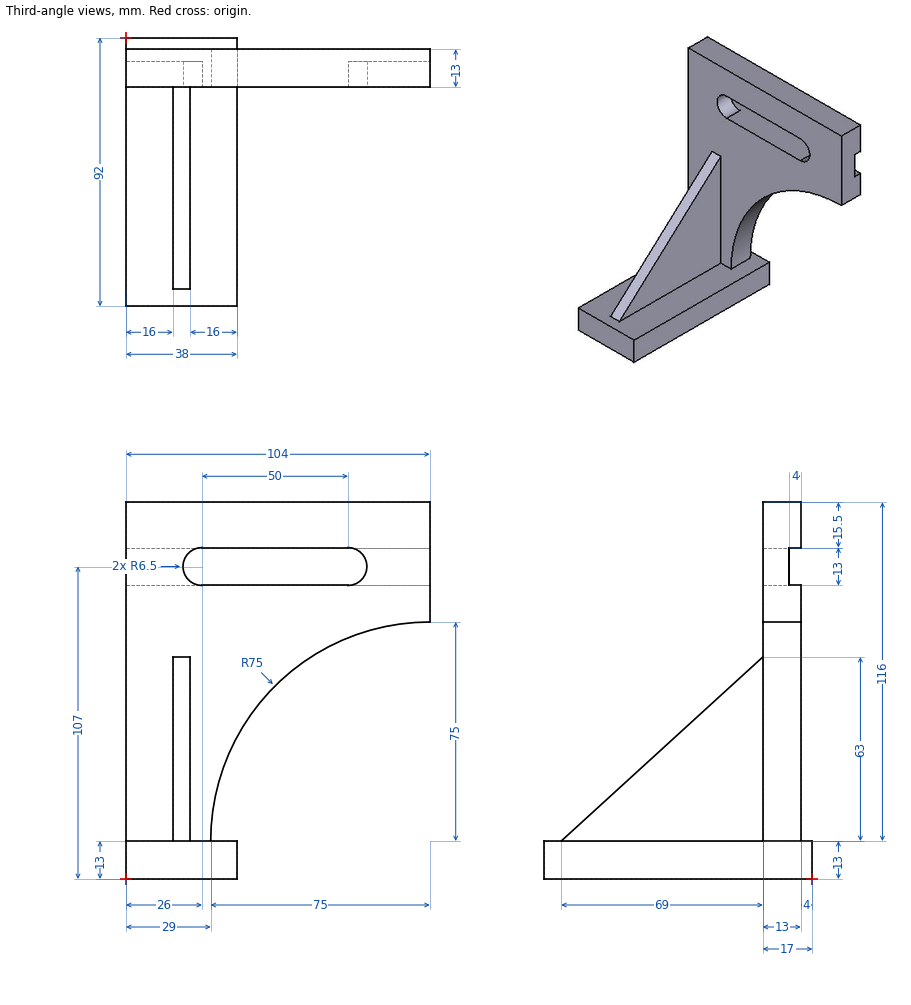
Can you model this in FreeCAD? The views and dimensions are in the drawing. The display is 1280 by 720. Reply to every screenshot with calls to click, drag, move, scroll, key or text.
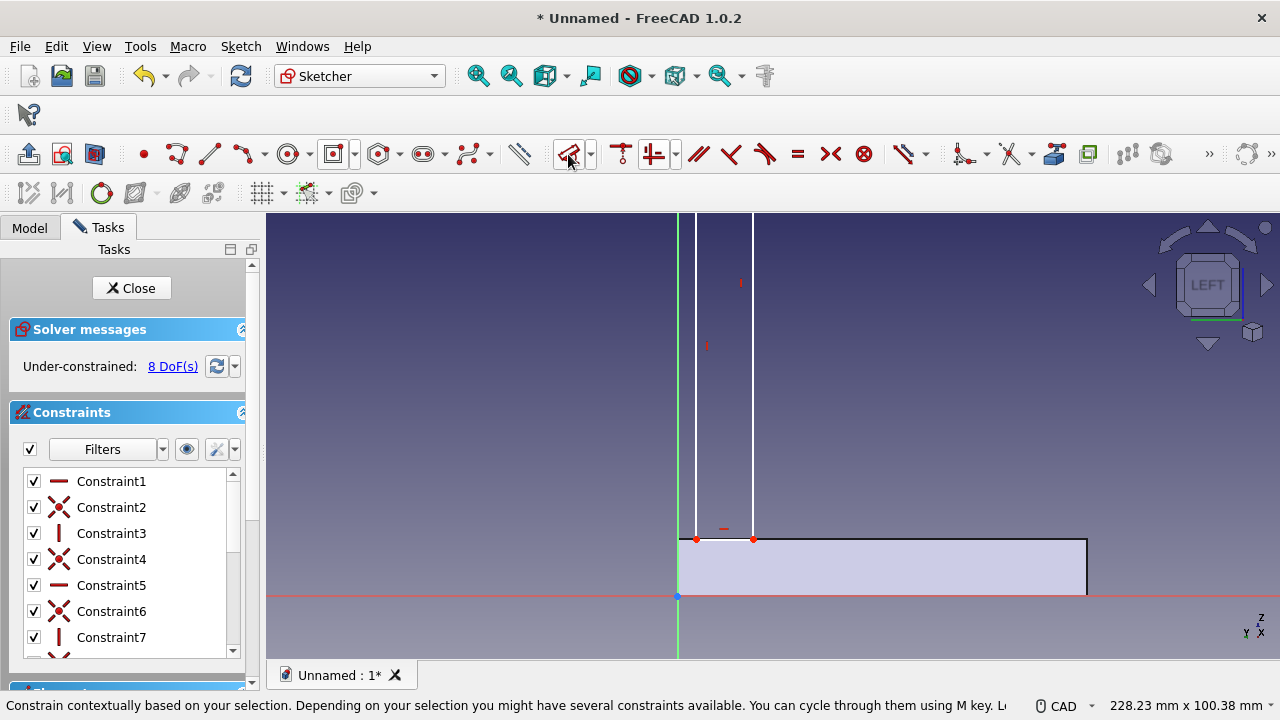
scroll(695, 539, down, 4)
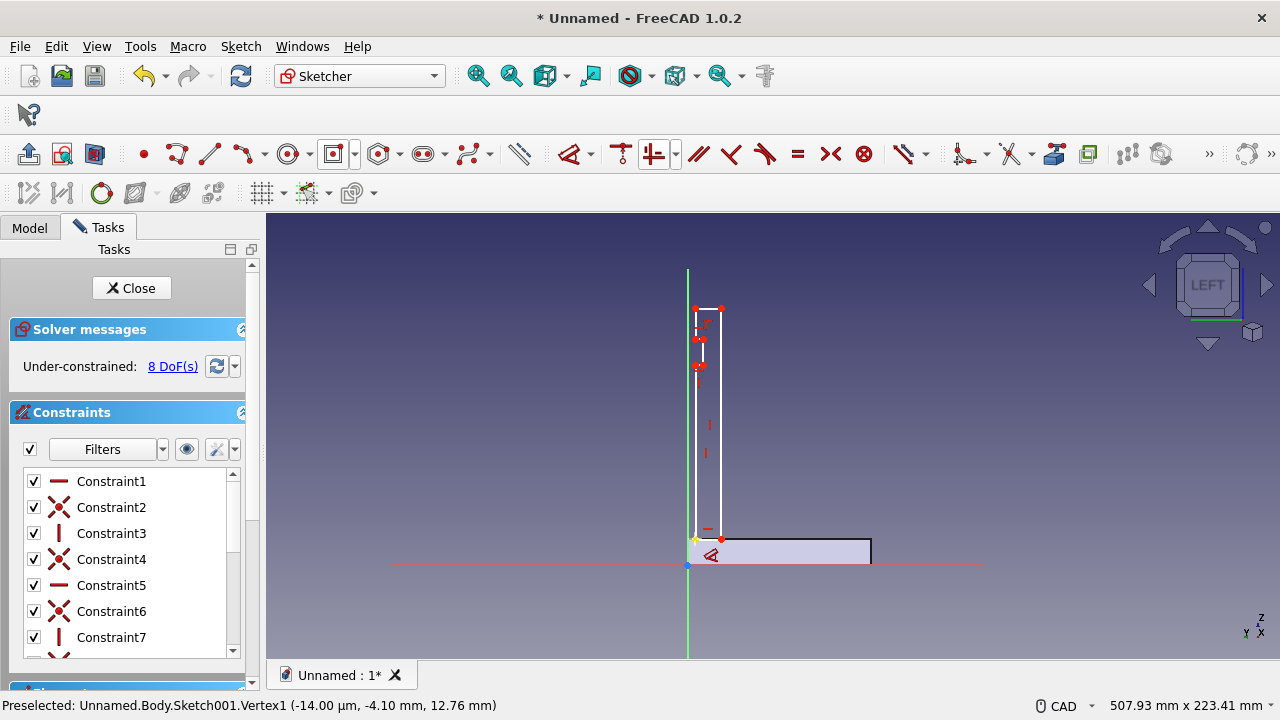
scroll(700, 339, up, 9)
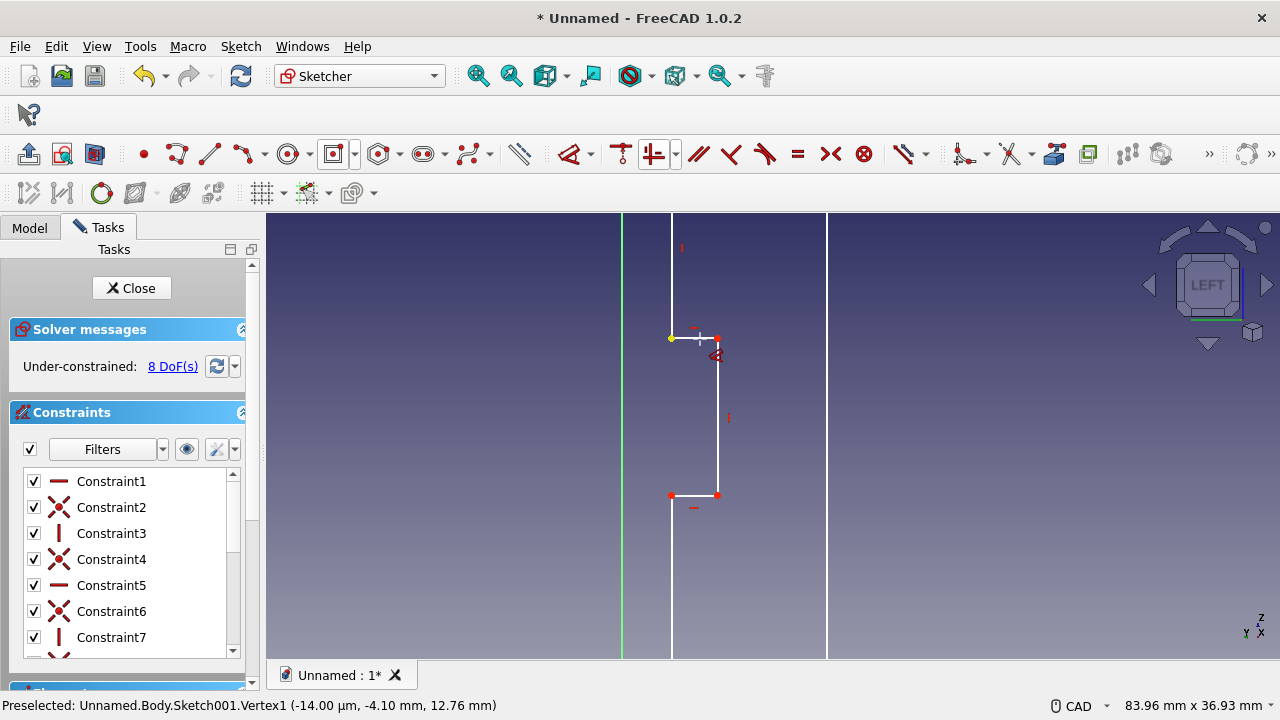
click(695, 338)
click(695, 304)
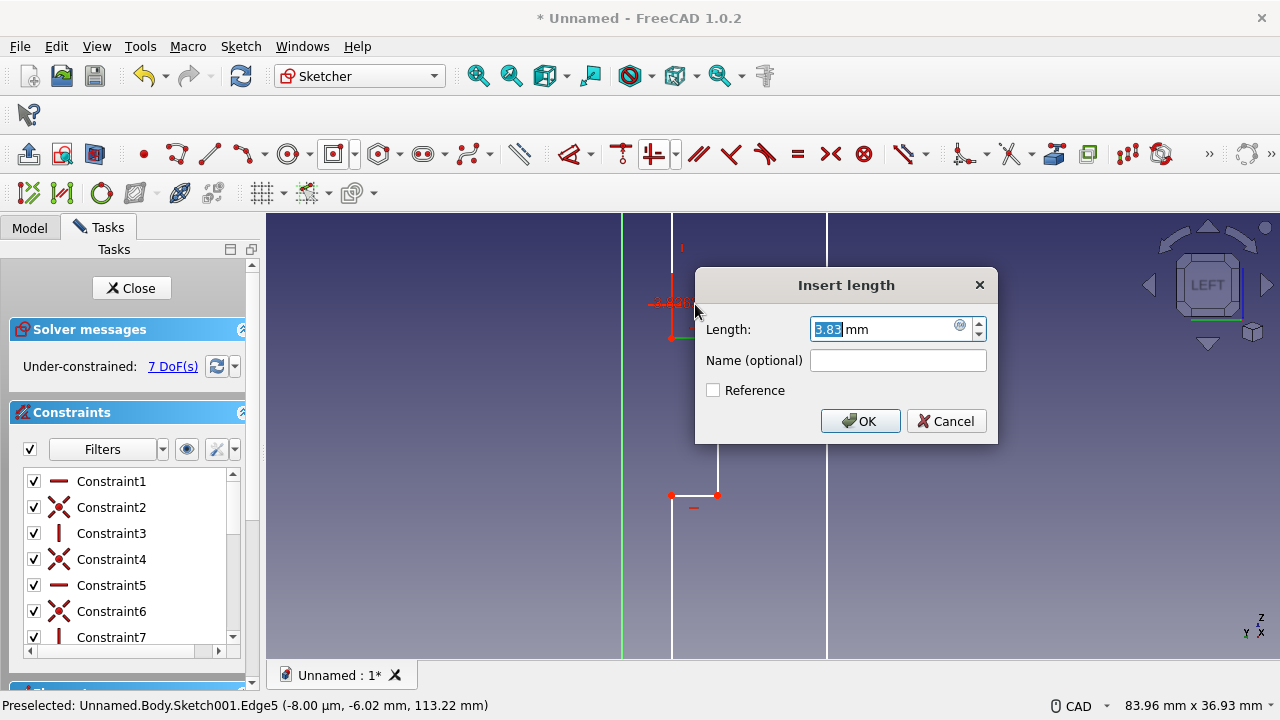
text(4)
key(Return)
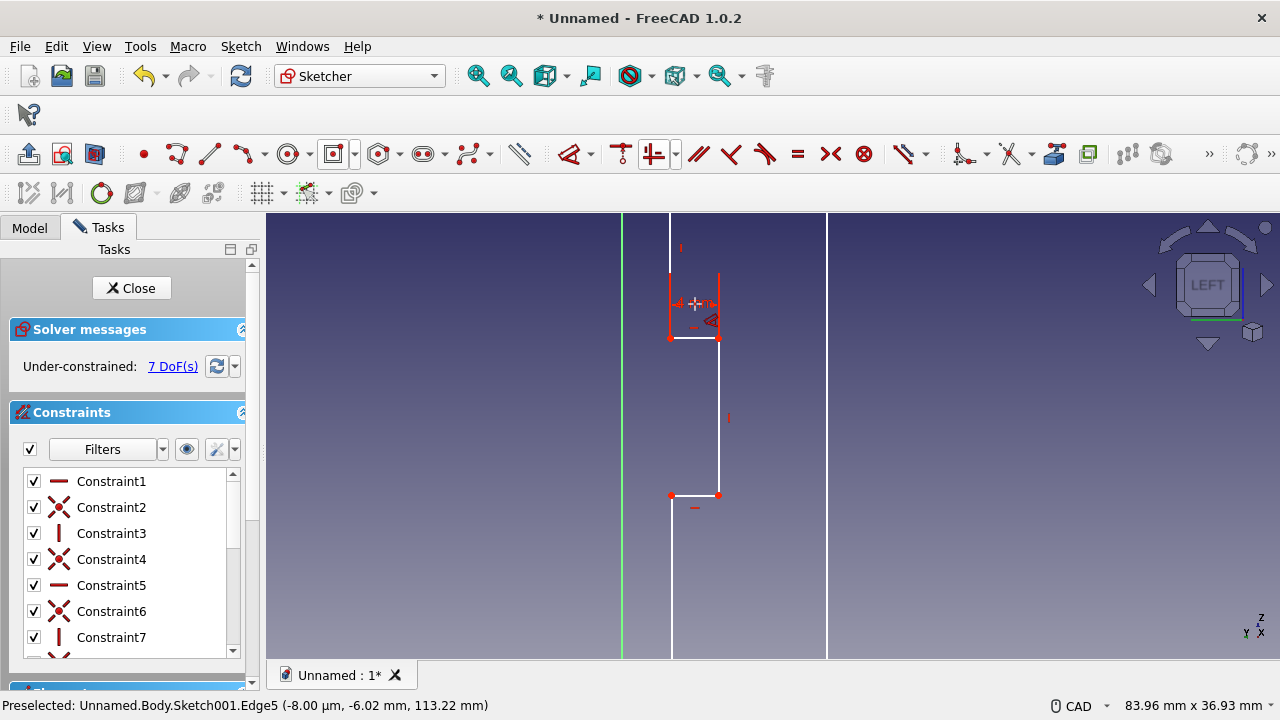
click(705, 496)
click(695, 462)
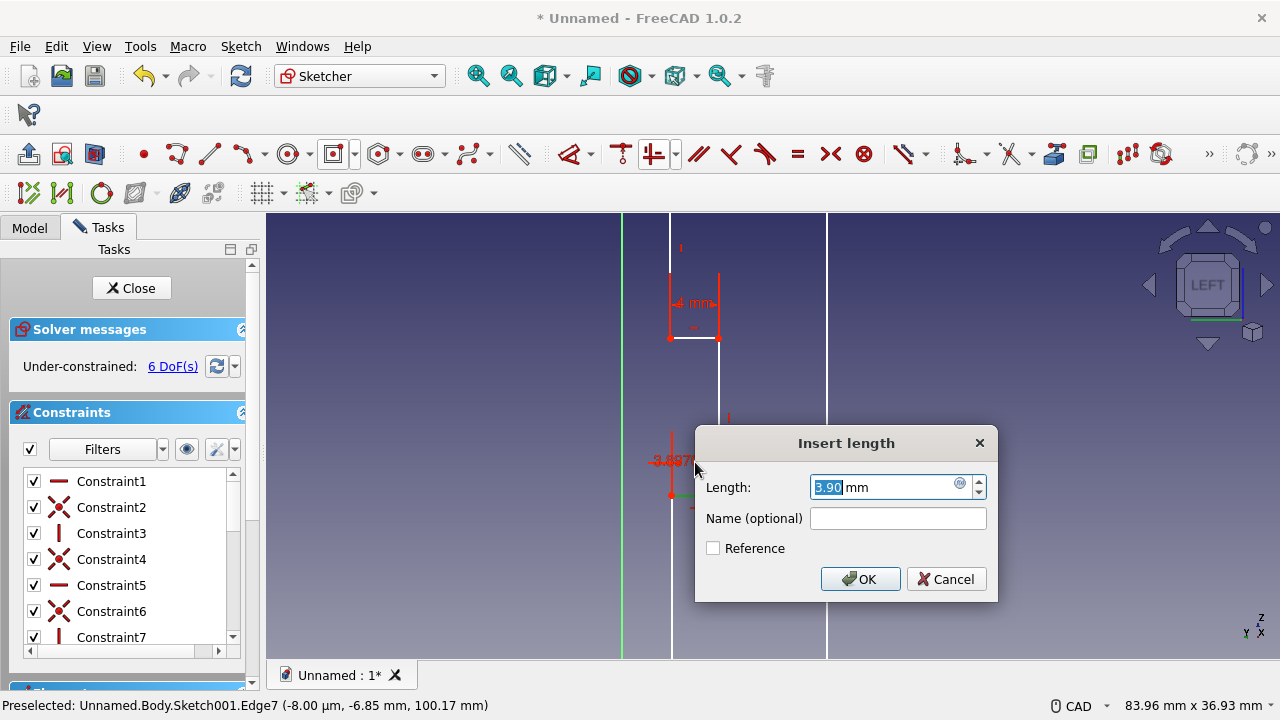
text(4)
key(Return)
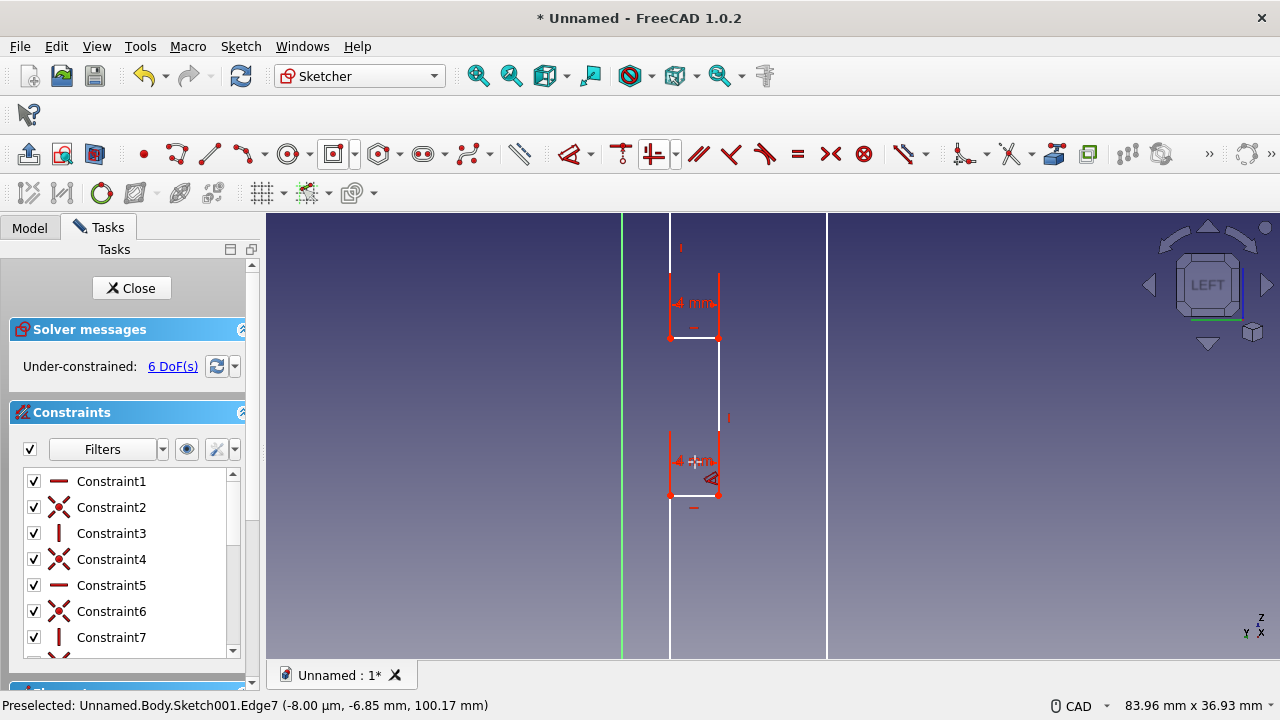
scroll(700, 339, down, 9)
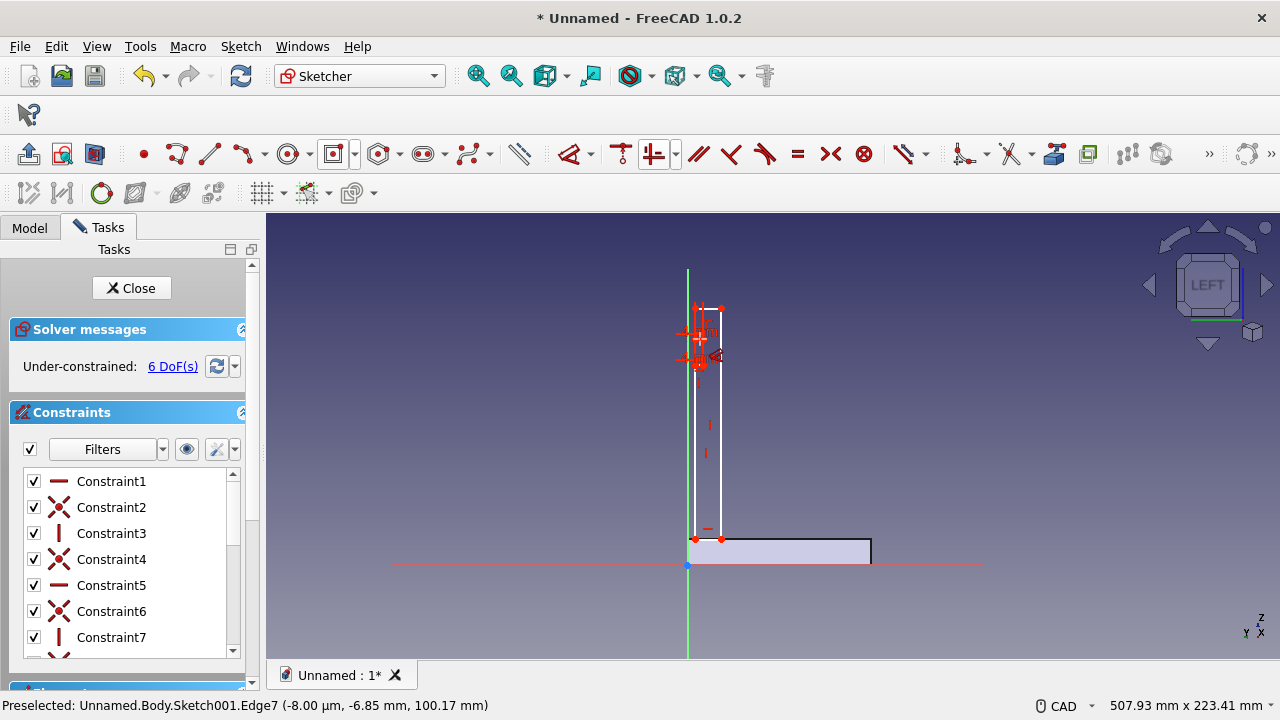
scroll(703, 540, up, 3)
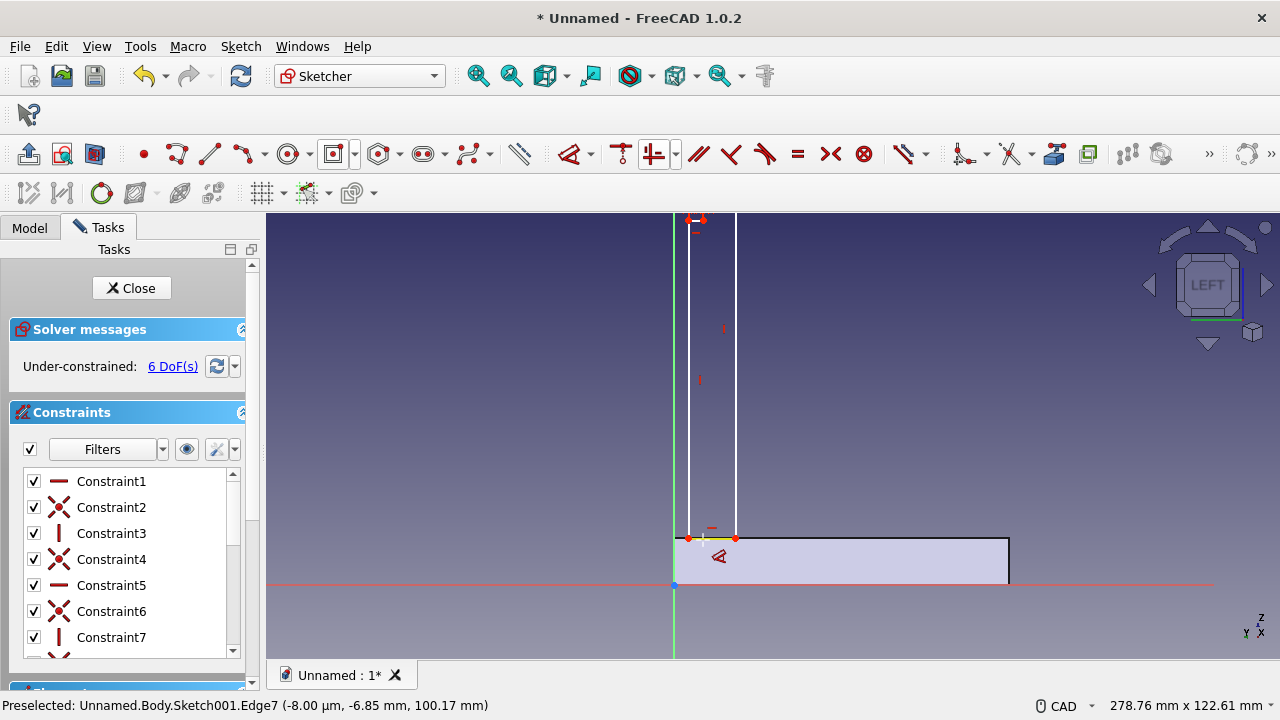
click(703, 539)
click(712, 505)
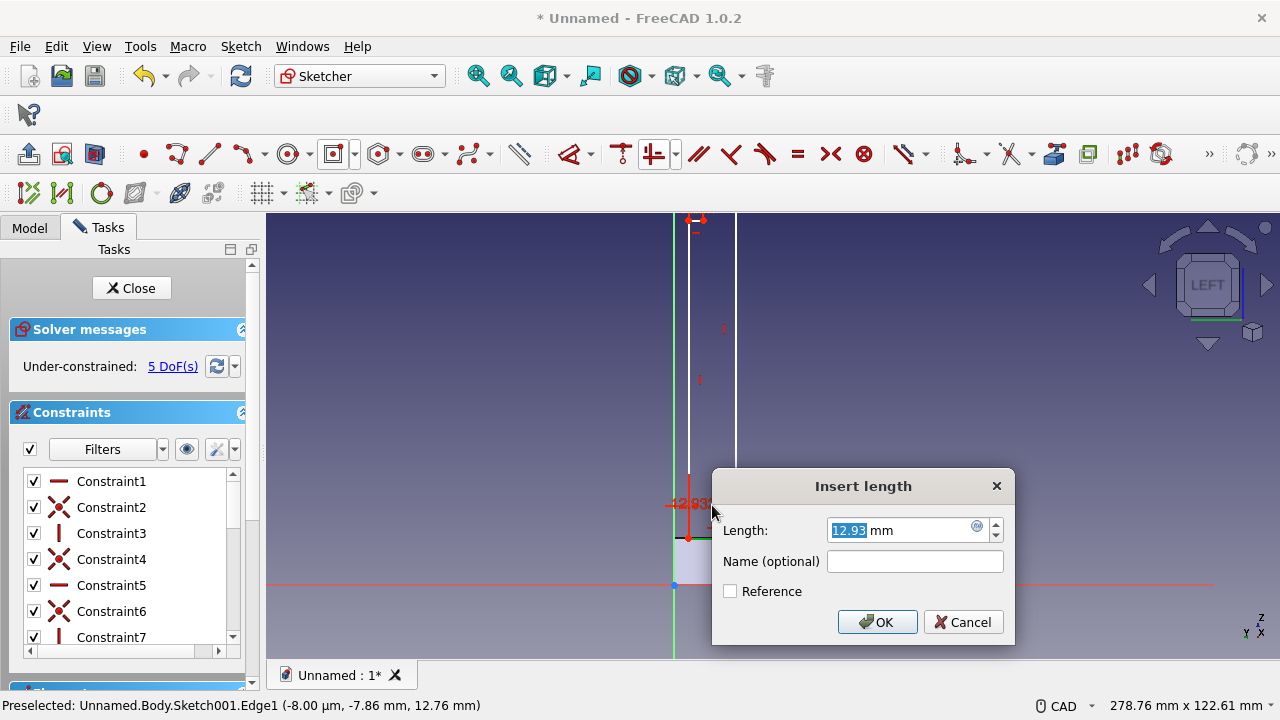
text(13)
key(Return)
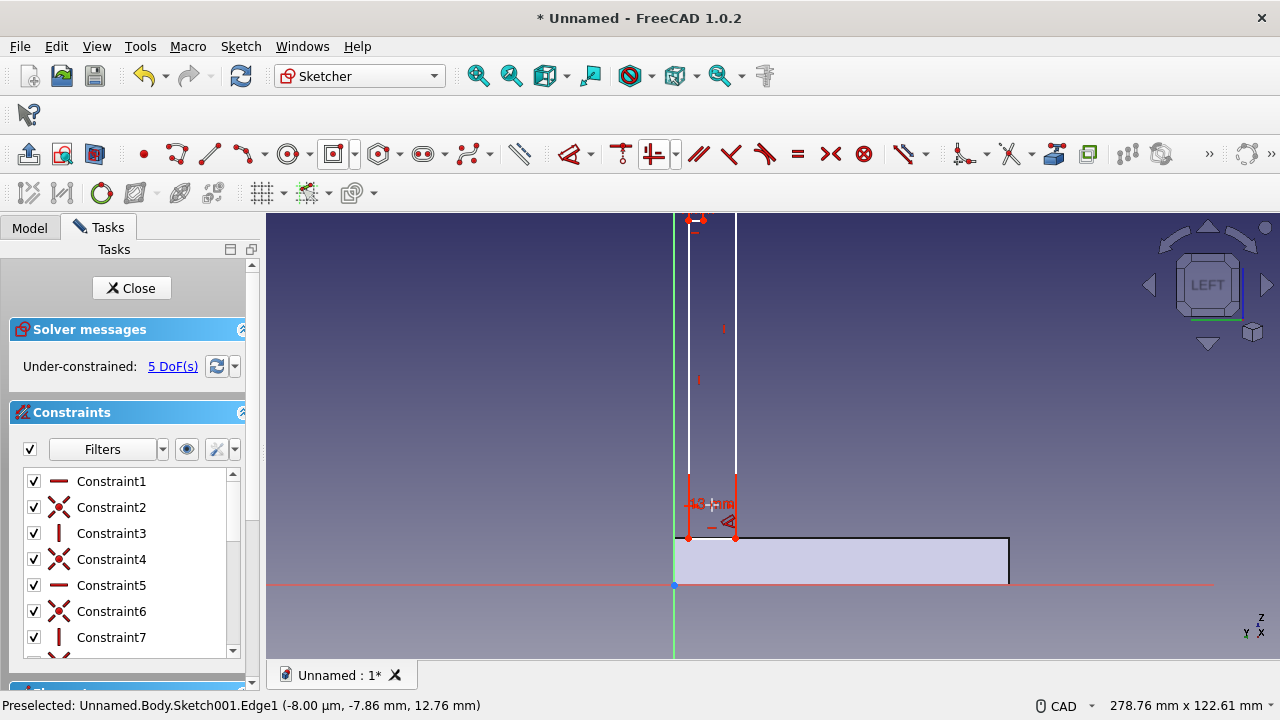
scroll(703, 540, down, 3)